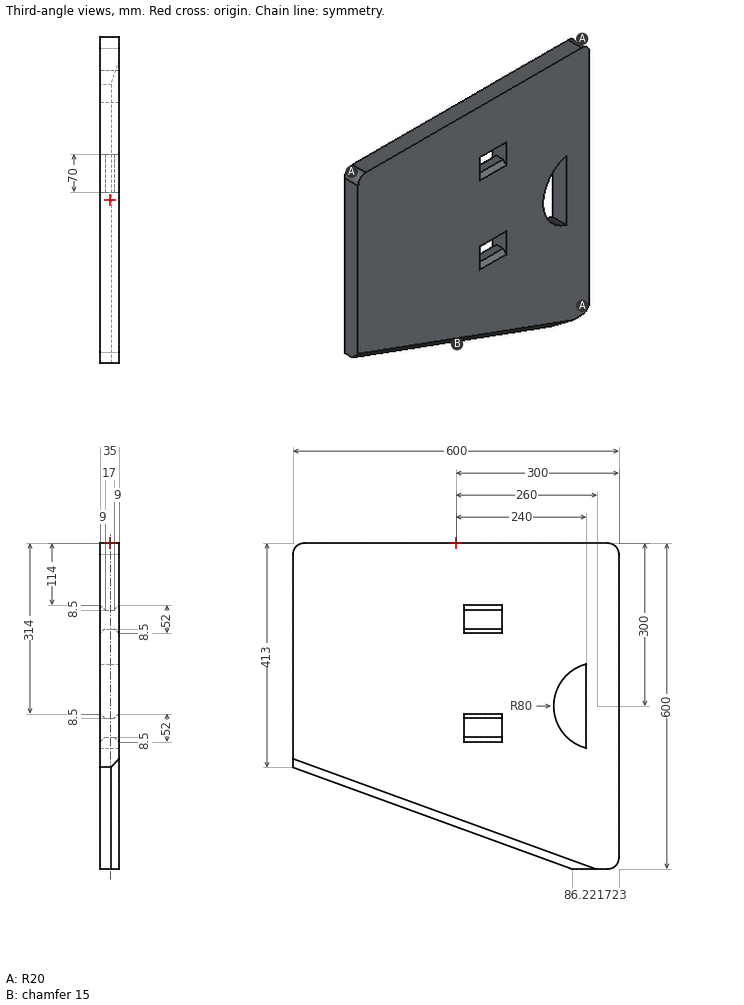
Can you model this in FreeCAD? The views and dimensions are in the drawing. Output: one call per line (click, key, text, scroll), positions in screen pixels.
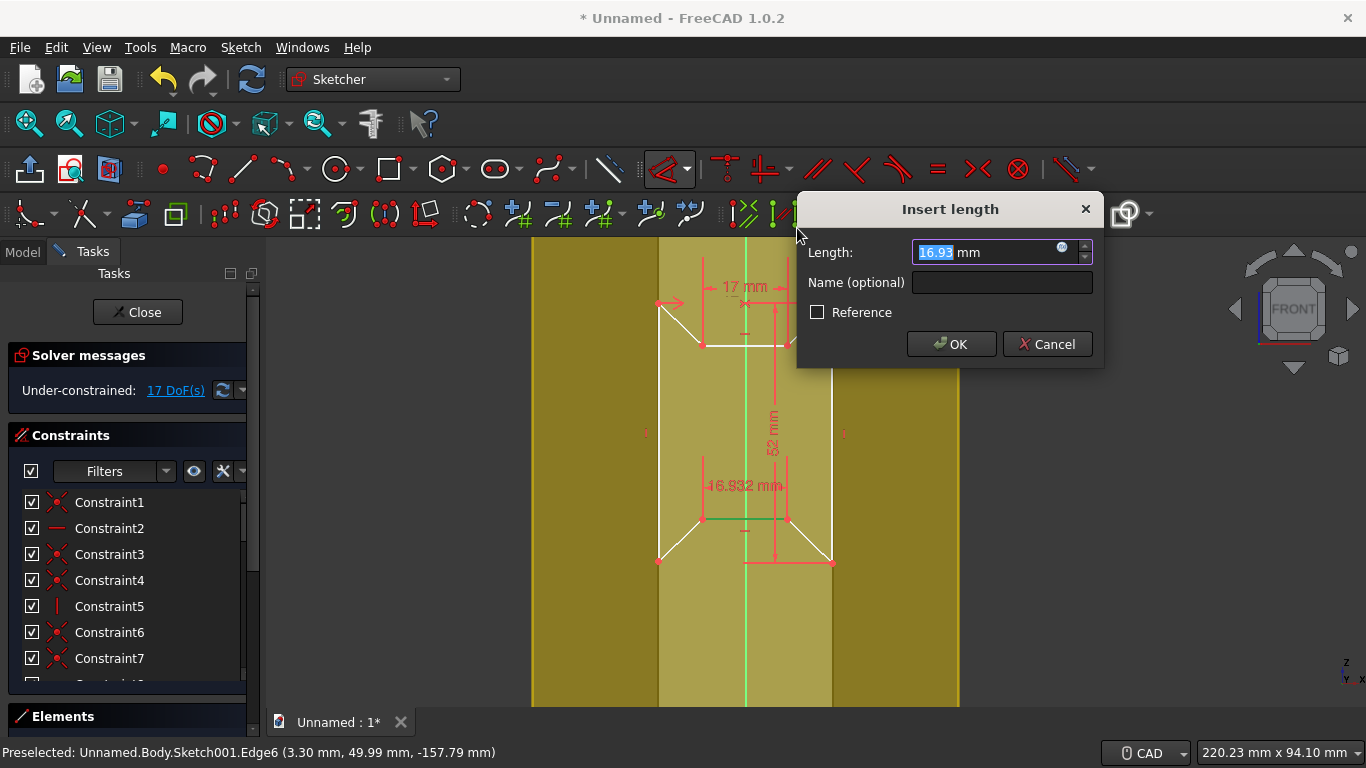
text(17)
key(Return)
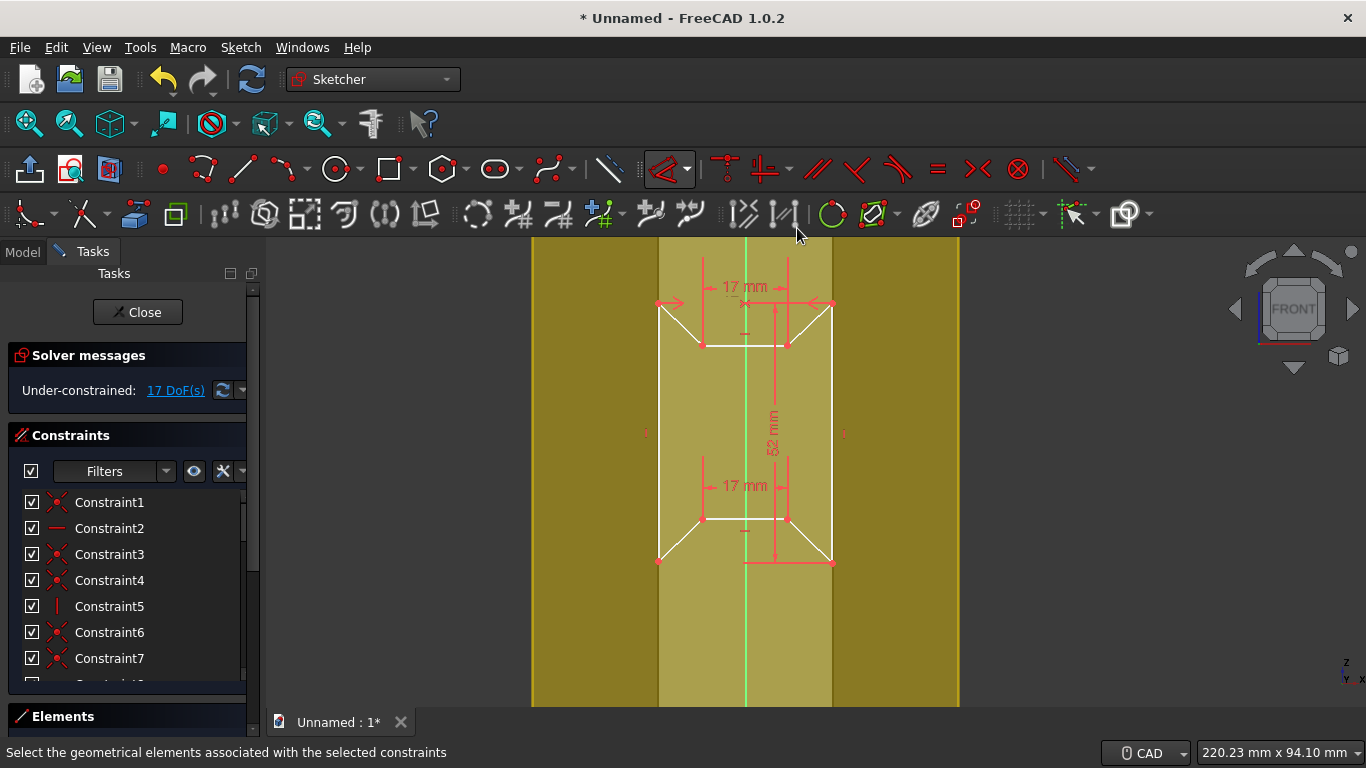
scroll(748, 438, down, 9)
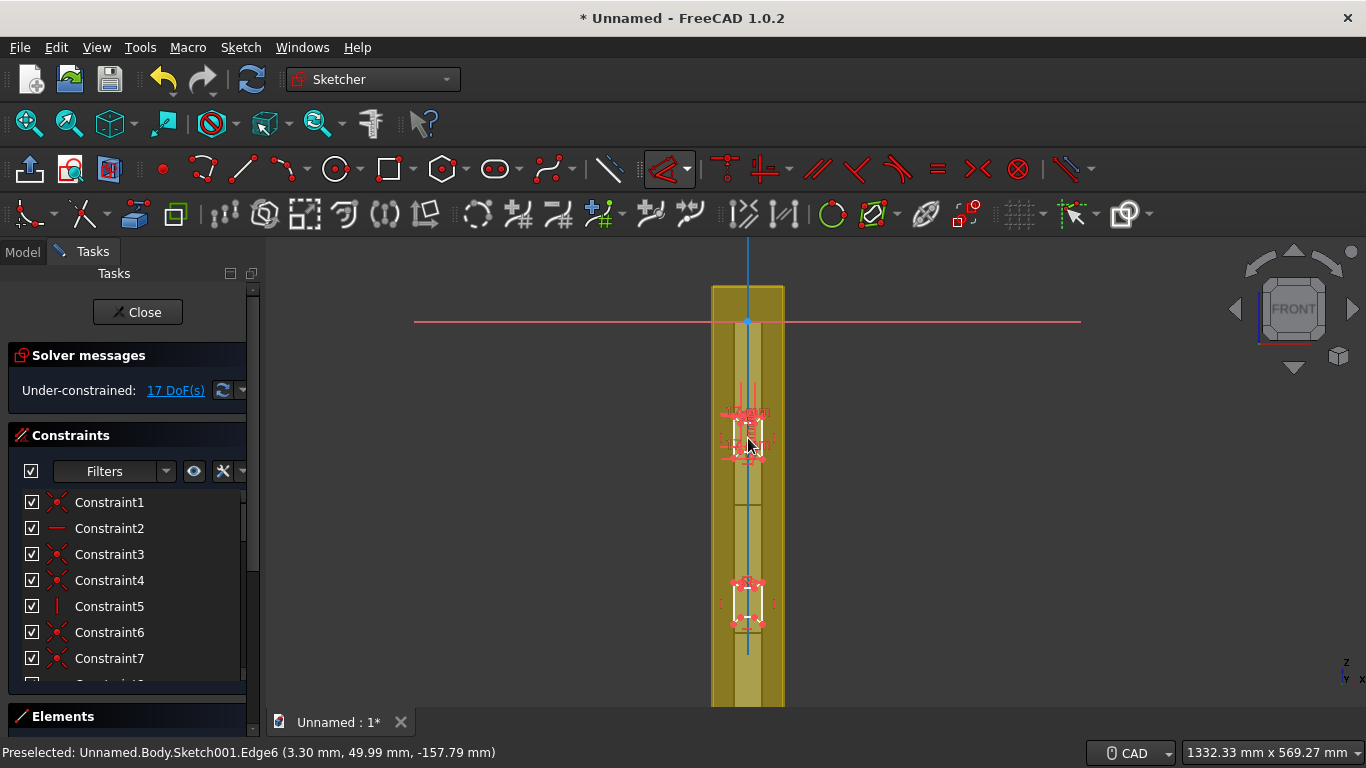
scroll(734, 446, up, 3)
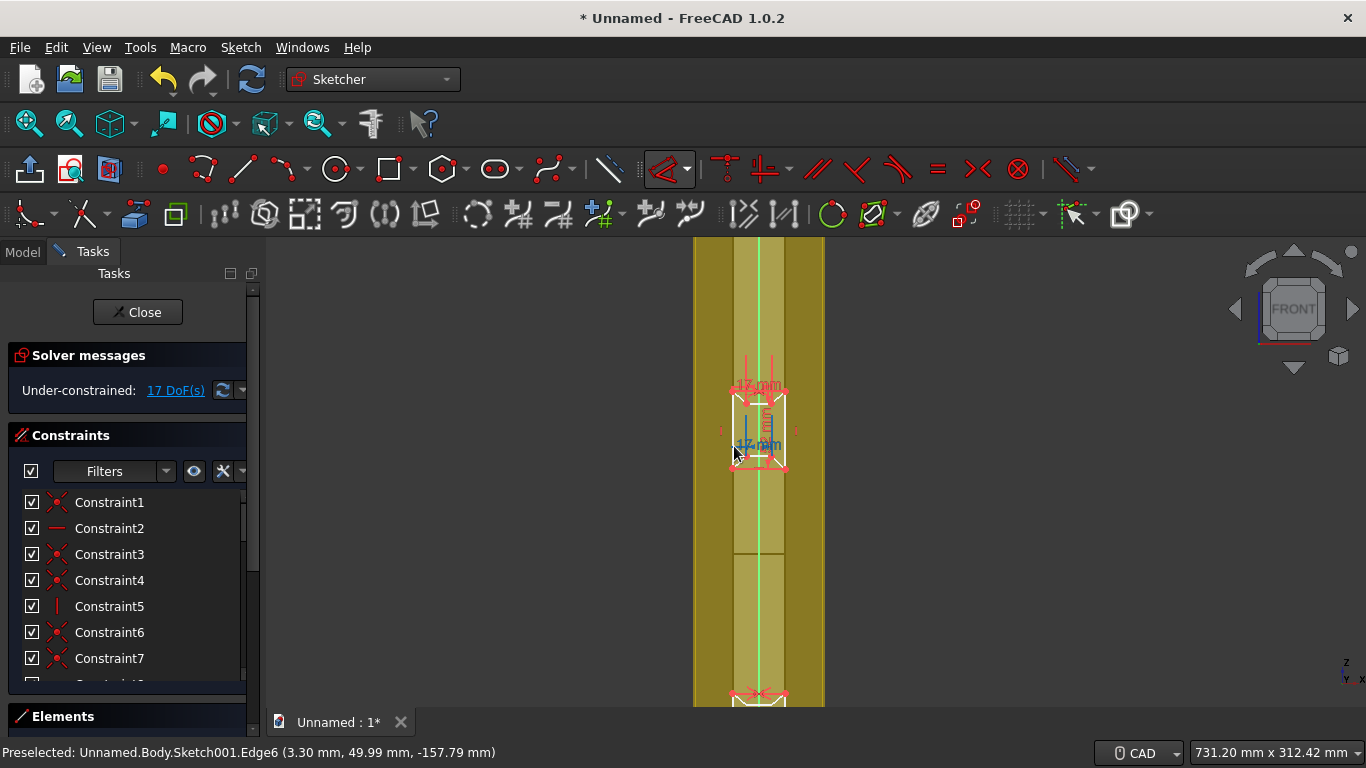
click(733, 446)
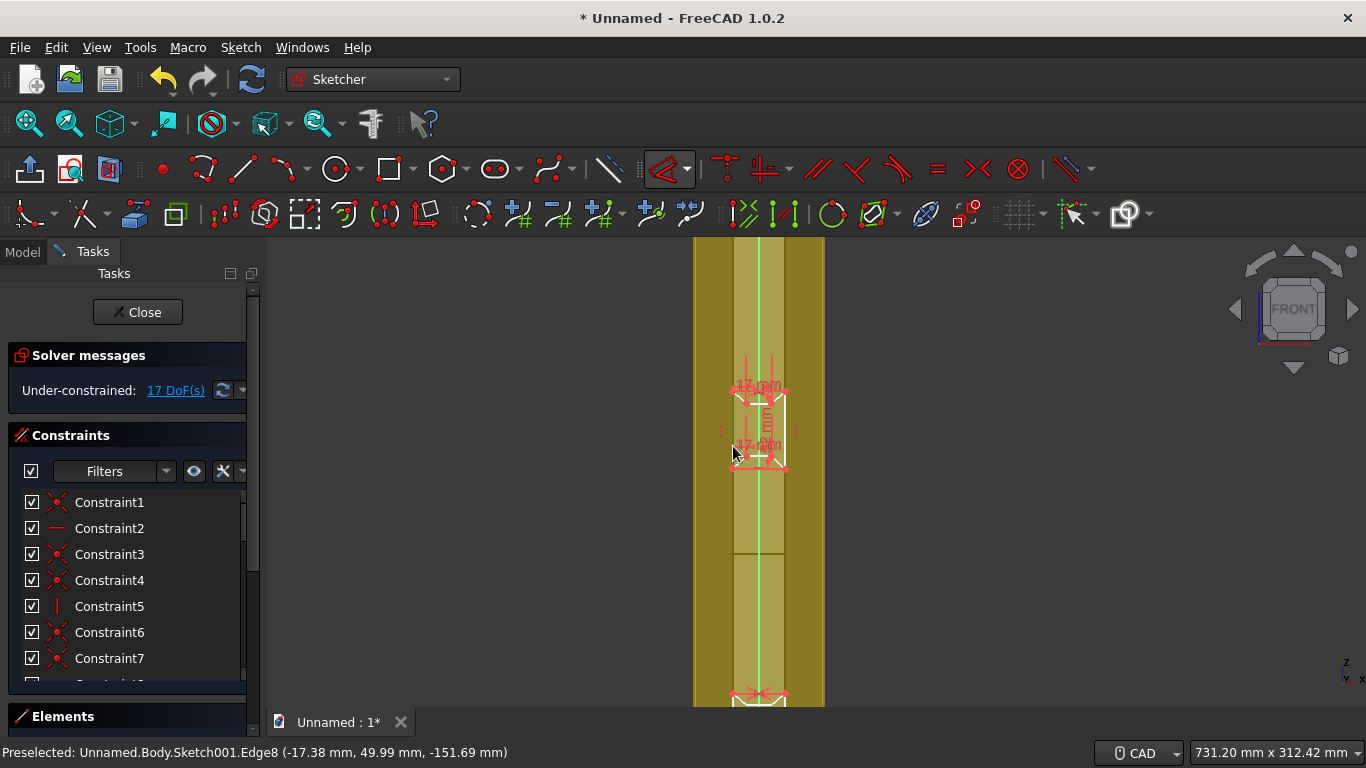
key(i)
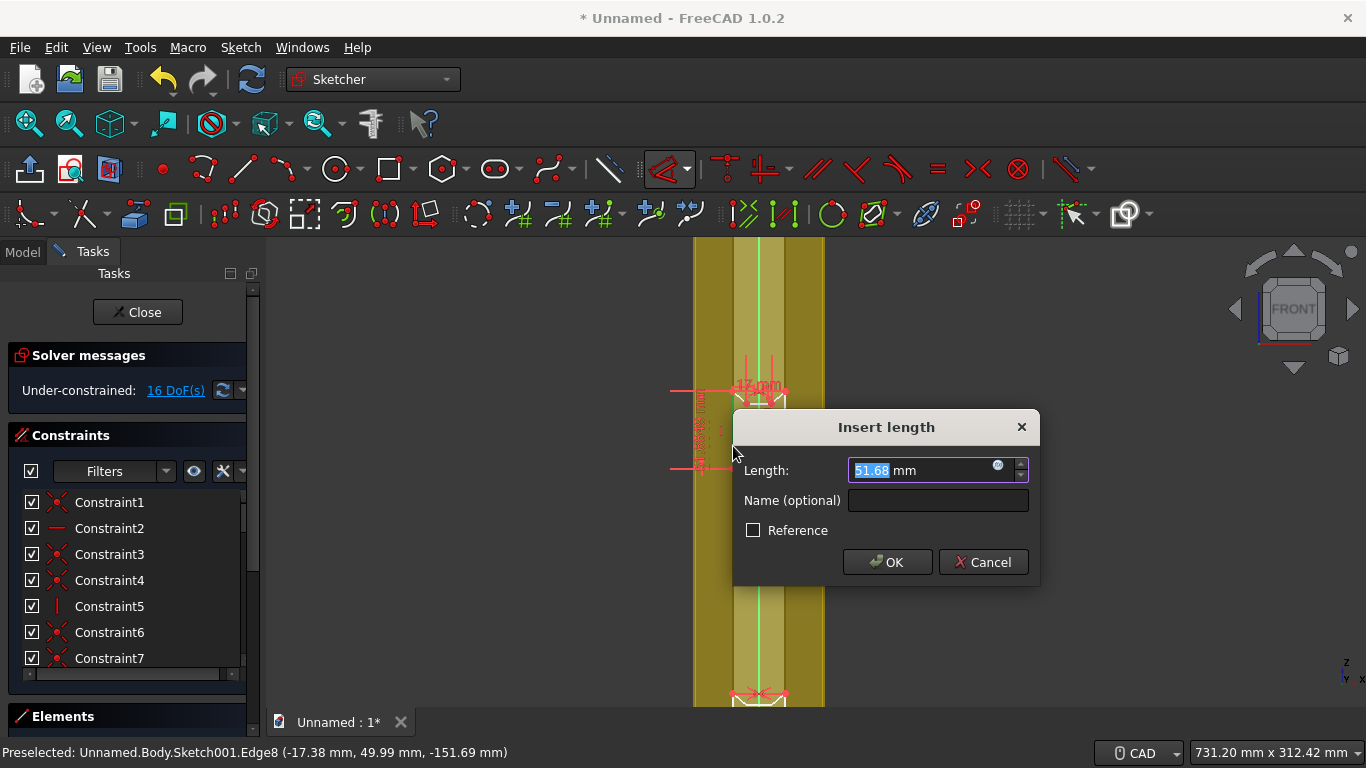
text(52)
key(Return)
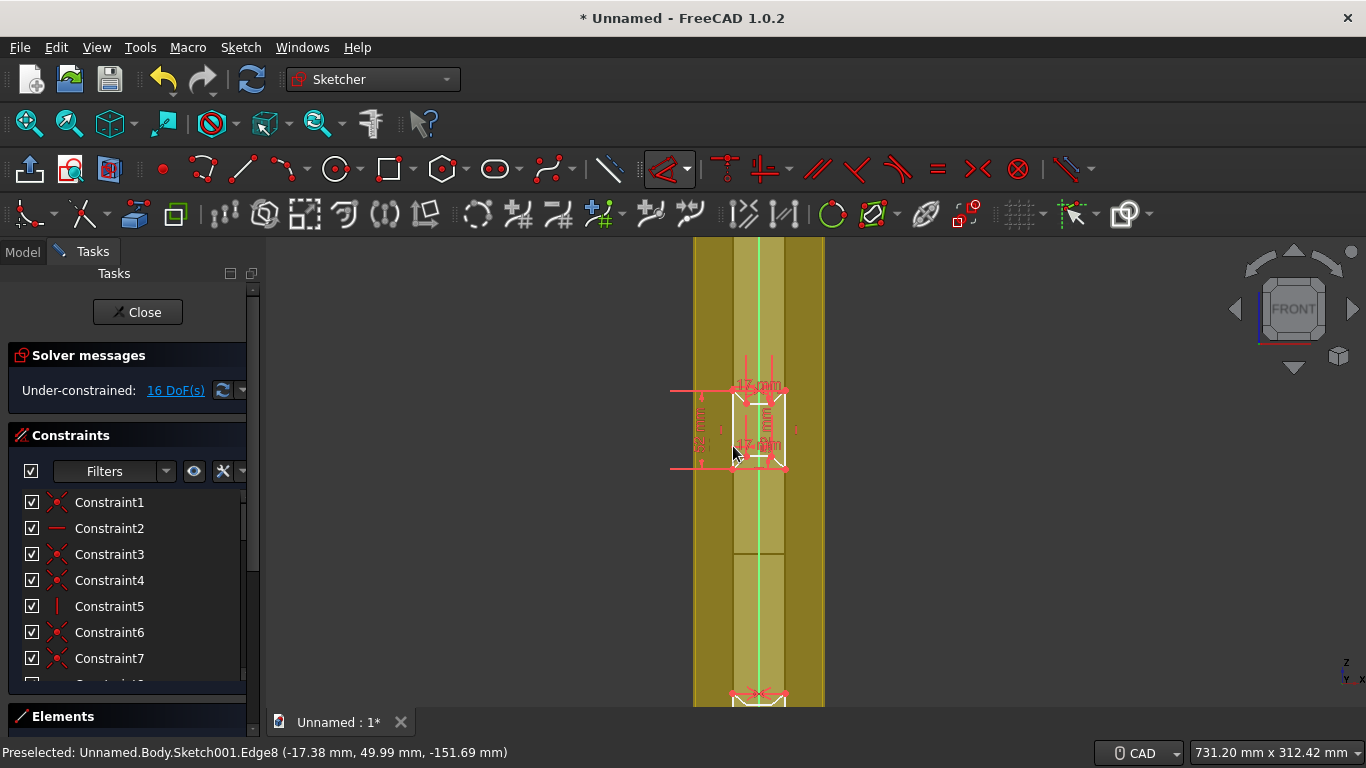
scroll(733, 445, down, 3)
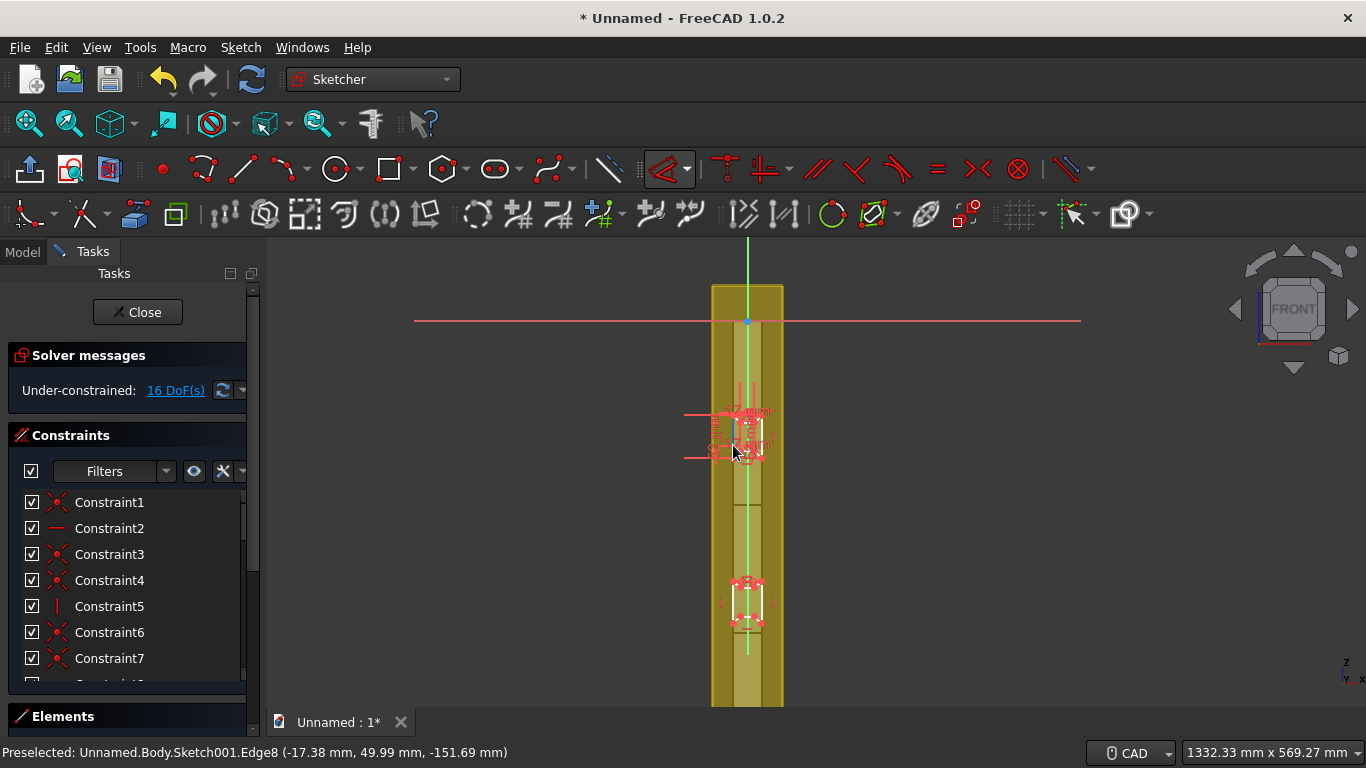
scroll(746, 588, up, 6)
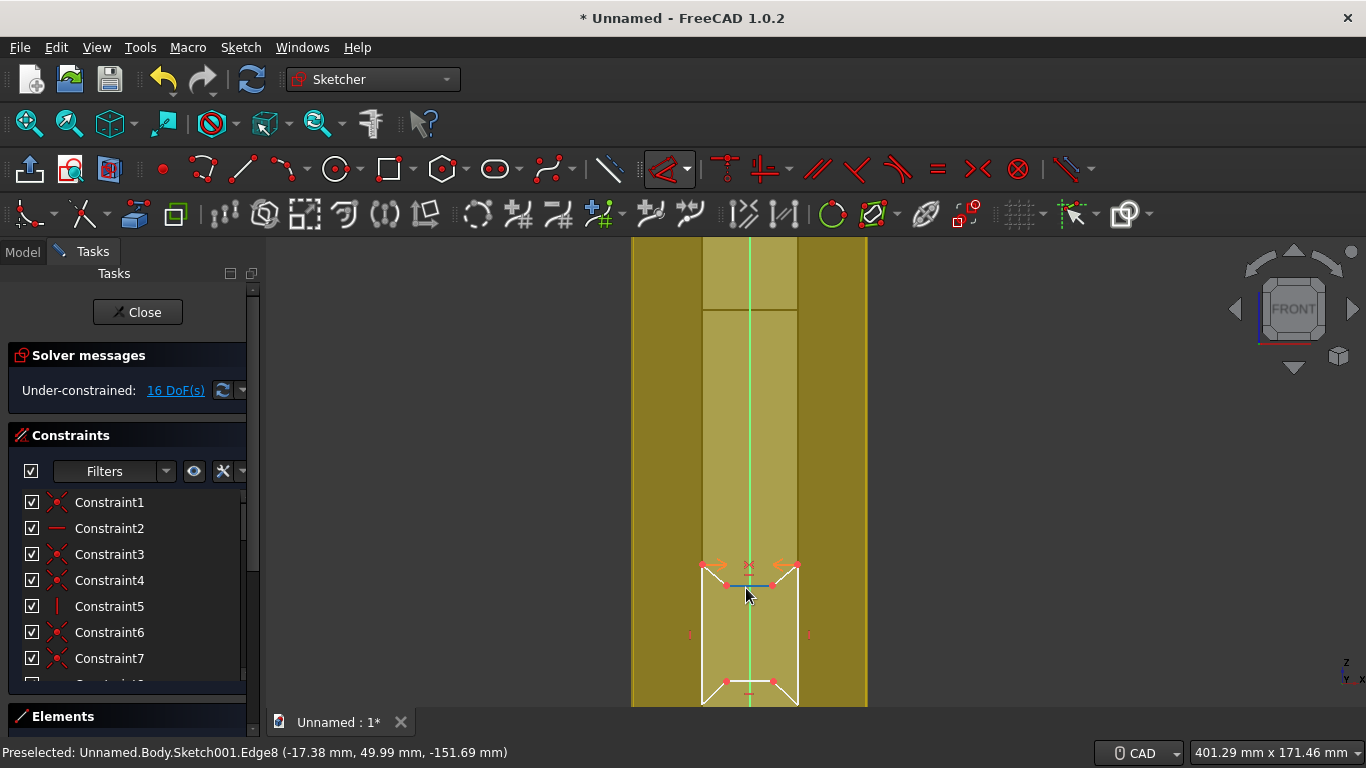
click(745, 586)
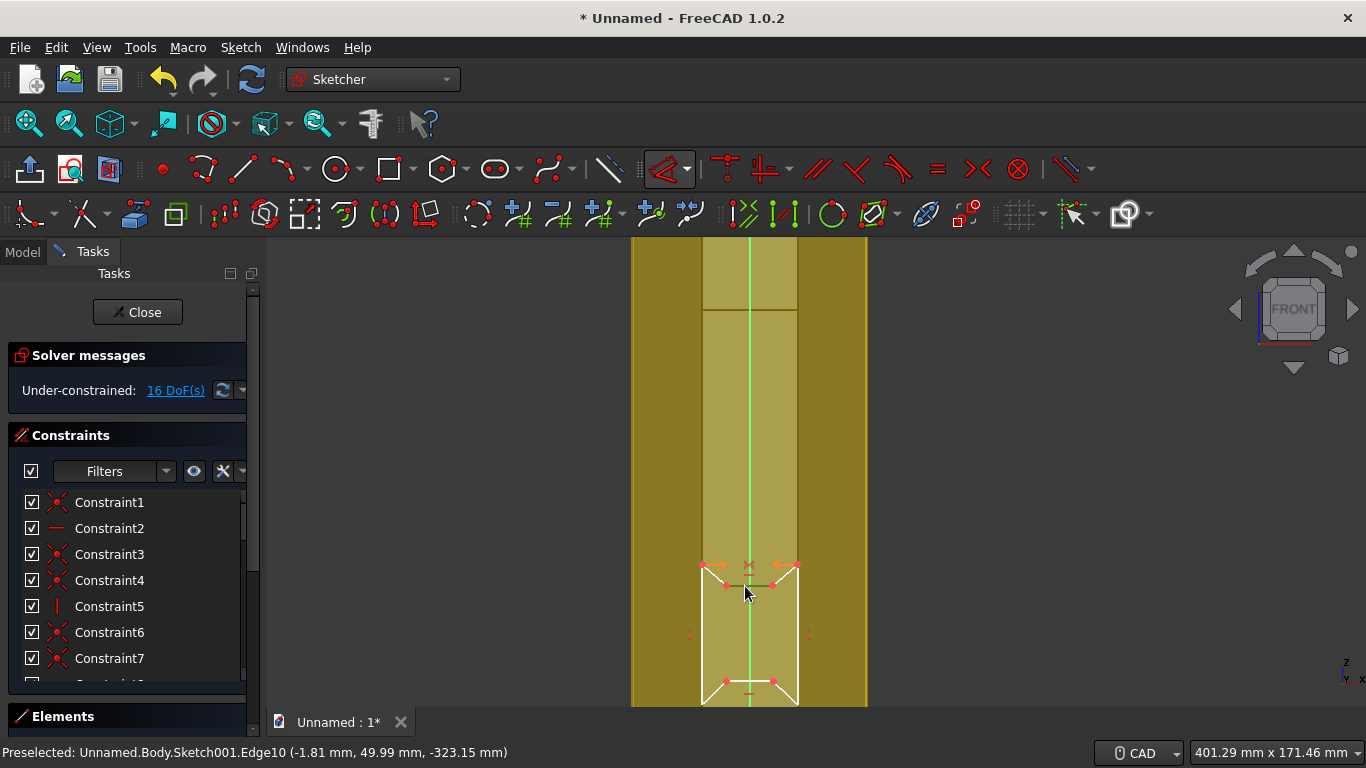
key(l)